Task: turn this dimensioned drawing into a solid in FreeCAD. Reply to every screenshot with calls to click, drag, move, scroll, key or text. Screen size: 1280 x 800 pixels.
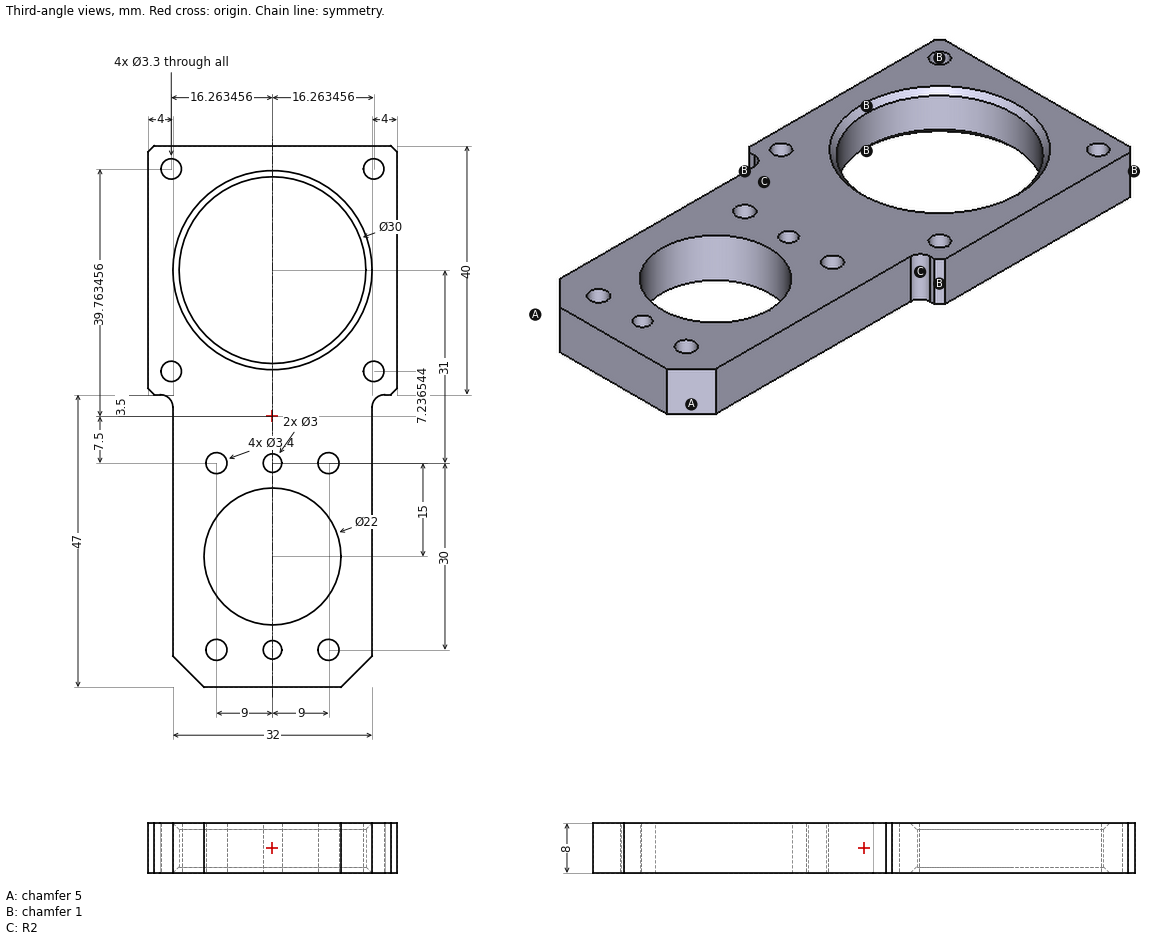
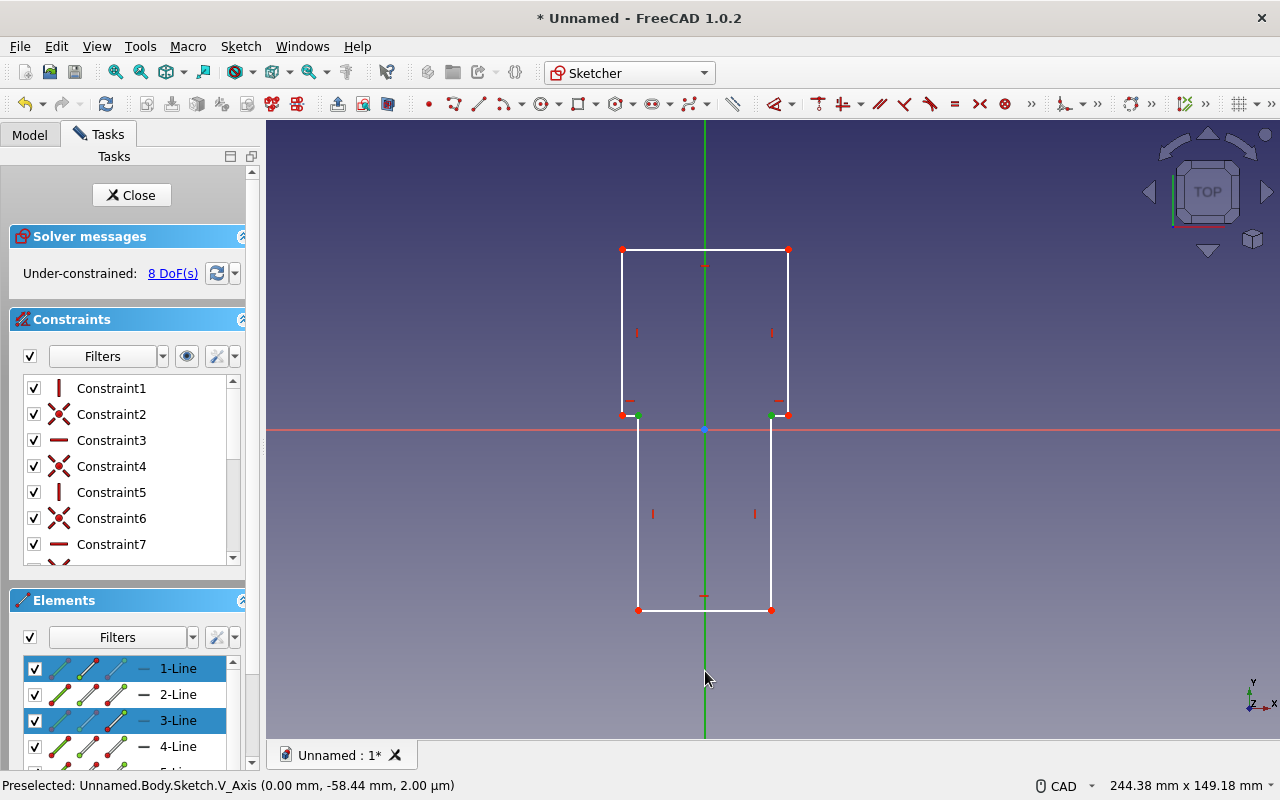
click(980, 104)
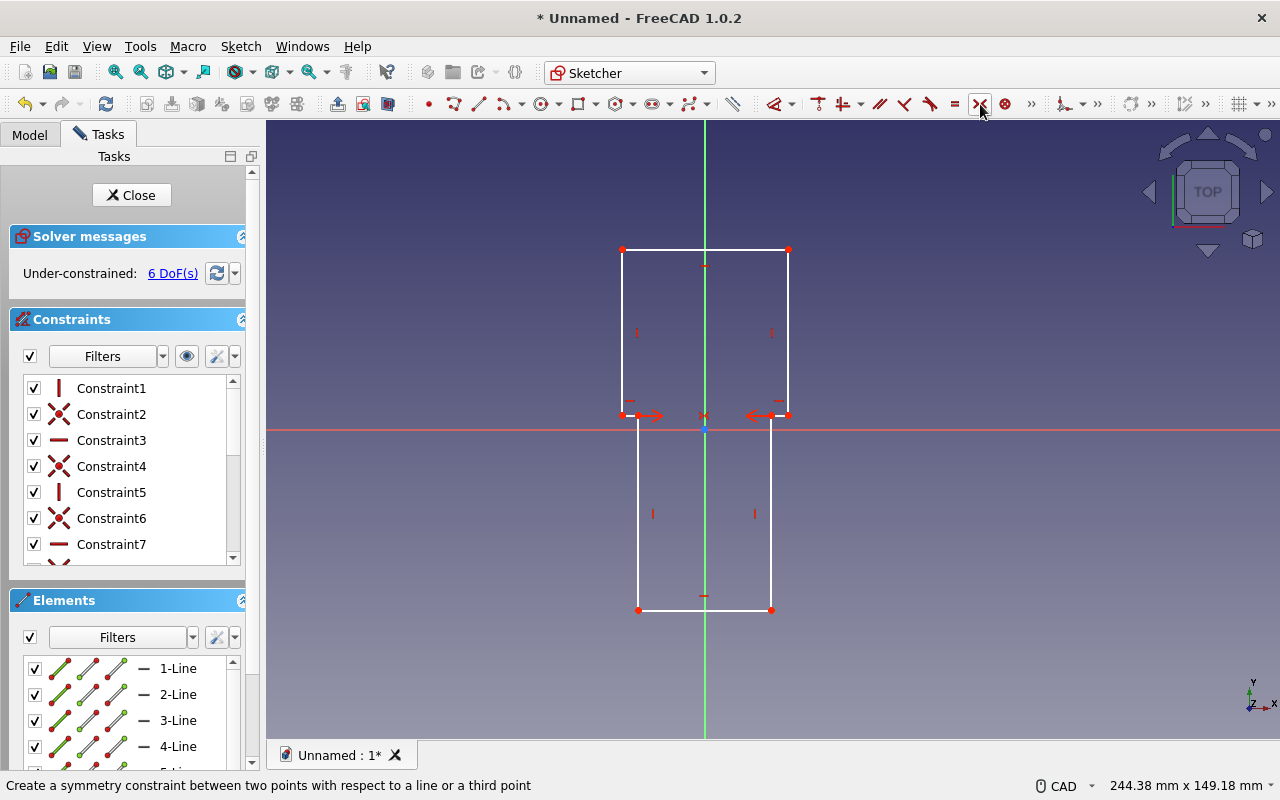
key(d)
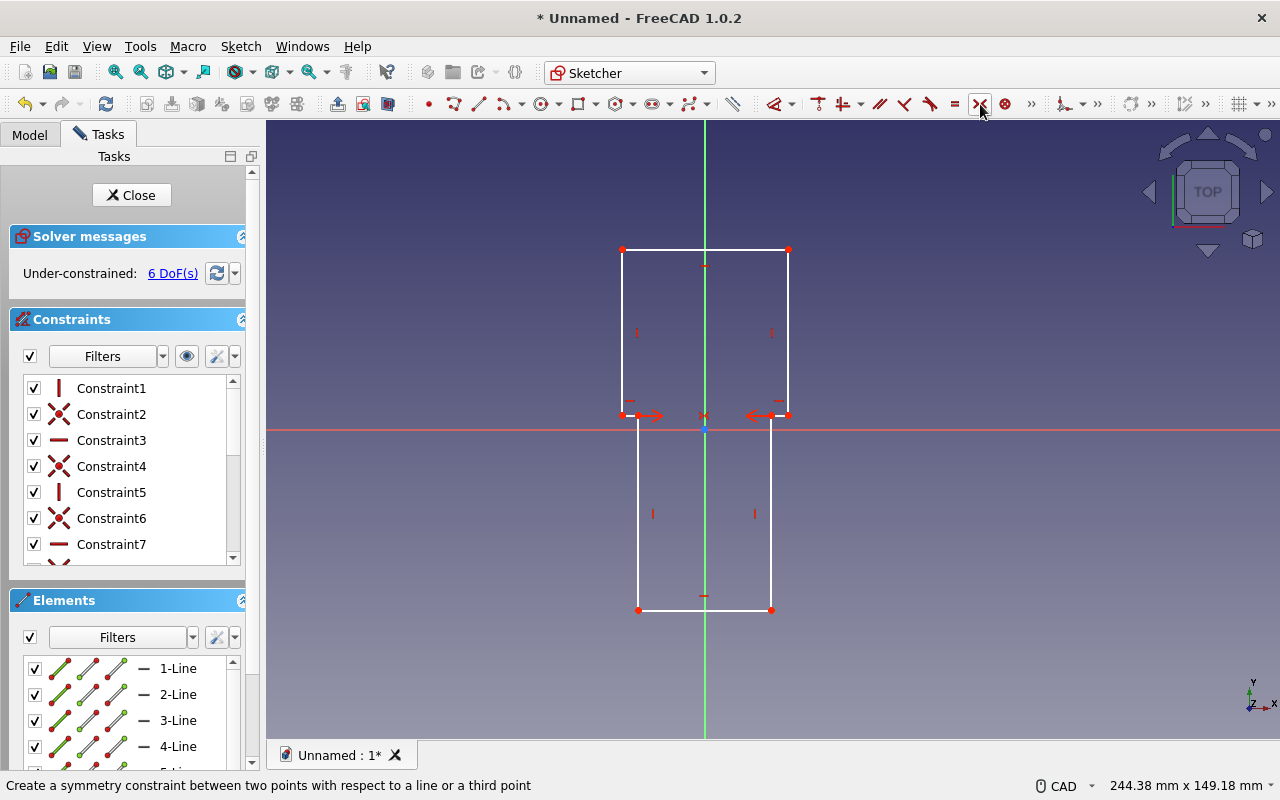
scroll(780, 416, up, 5)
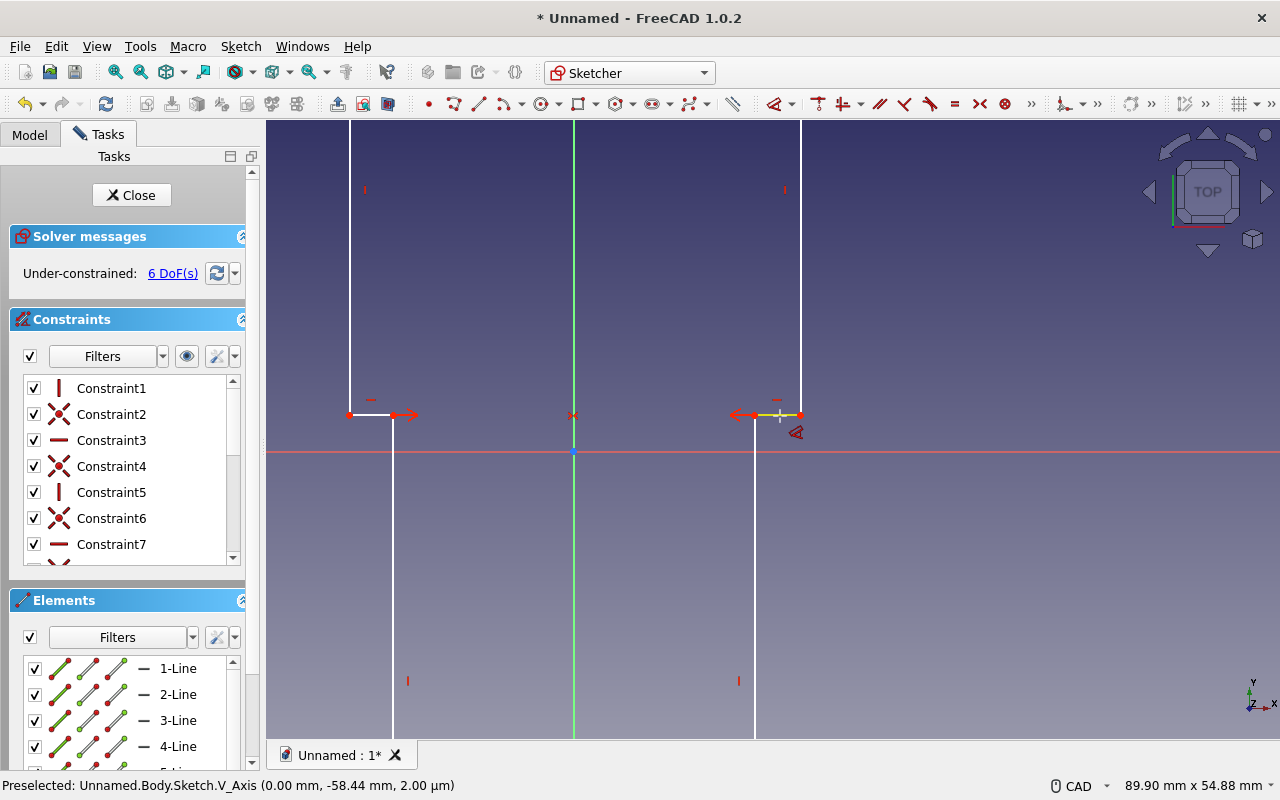
click(778, 415)
click(778, 381)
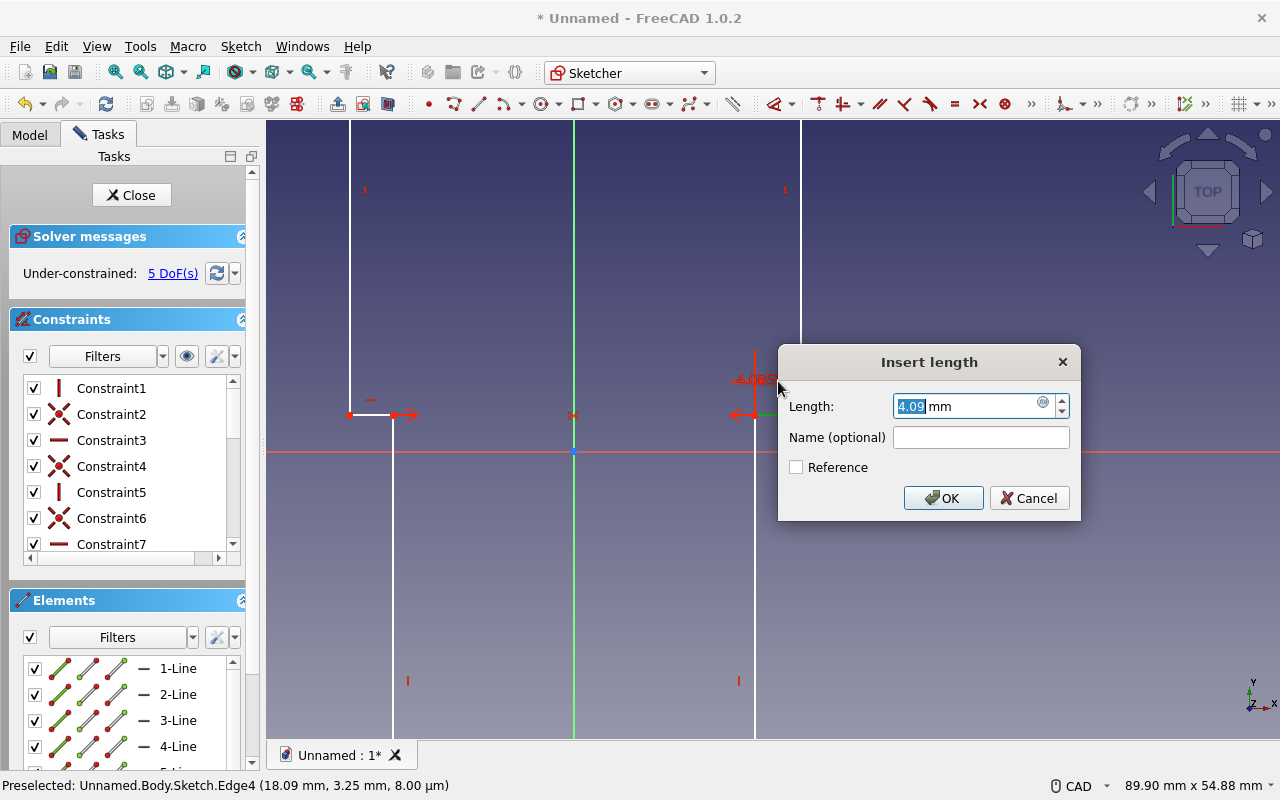
text(4)
key(Return)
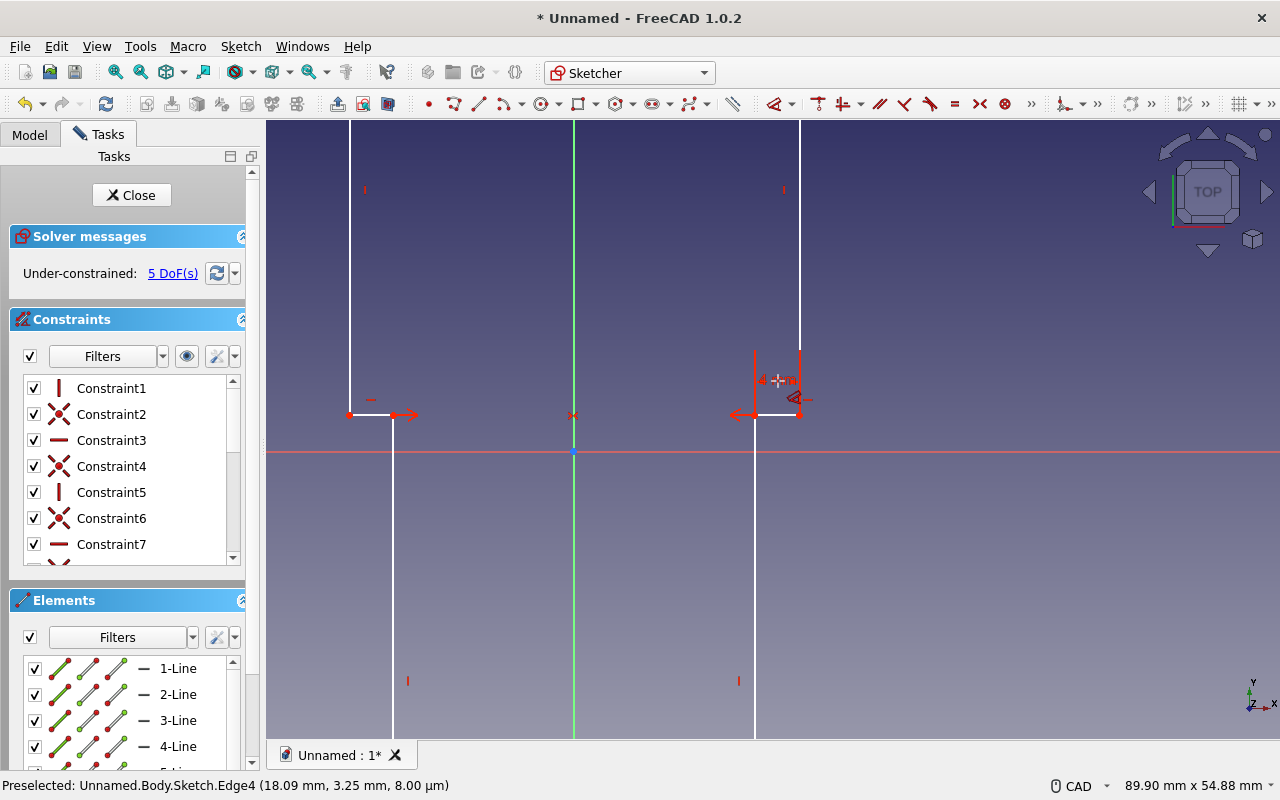
click(363, 415)
click(371, 381)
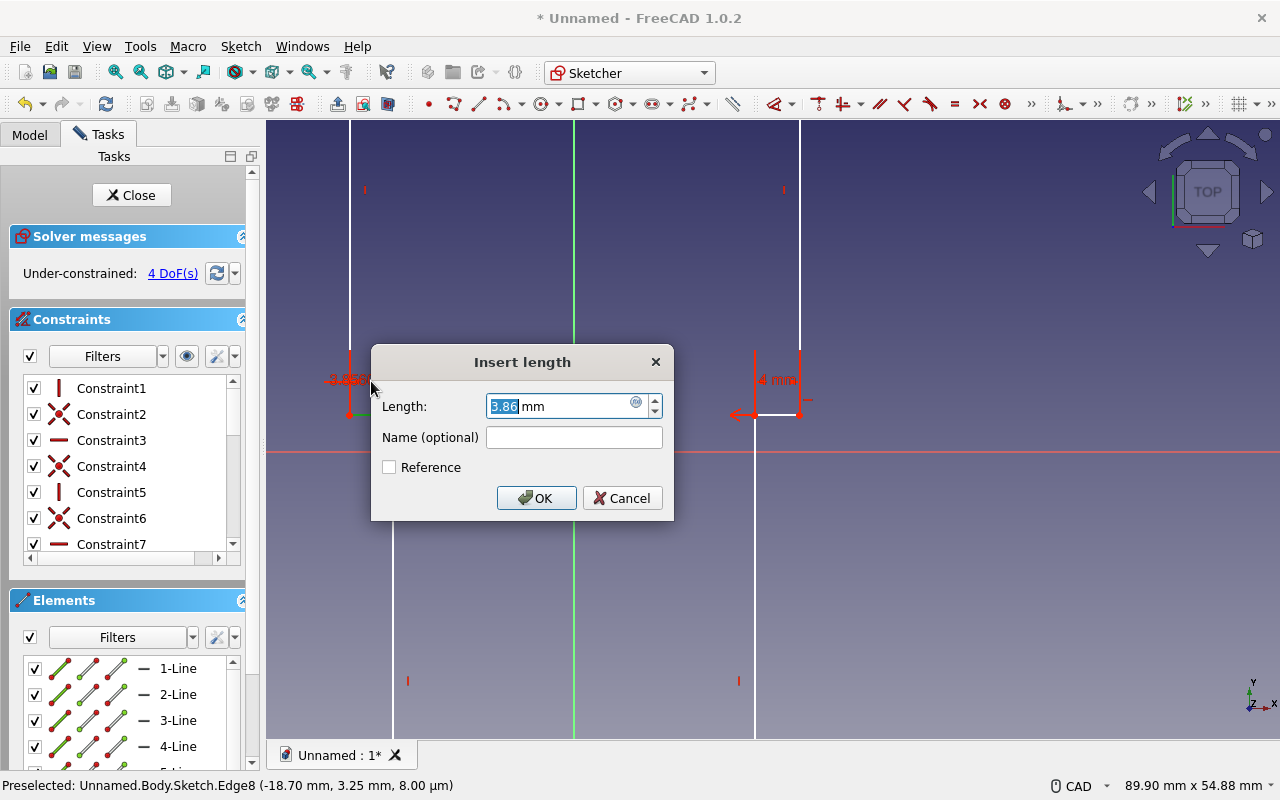
text(4)
key(Return)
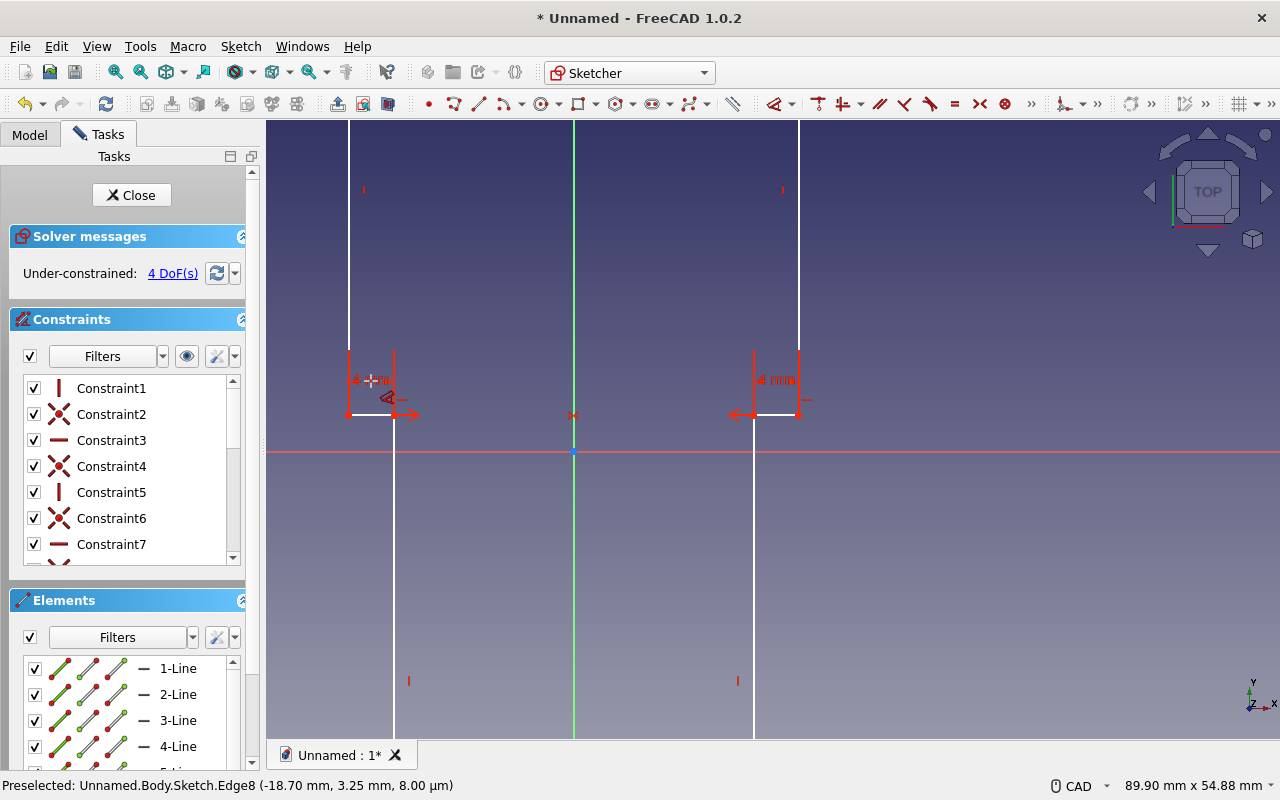
click(394, 574)
click(360, 563)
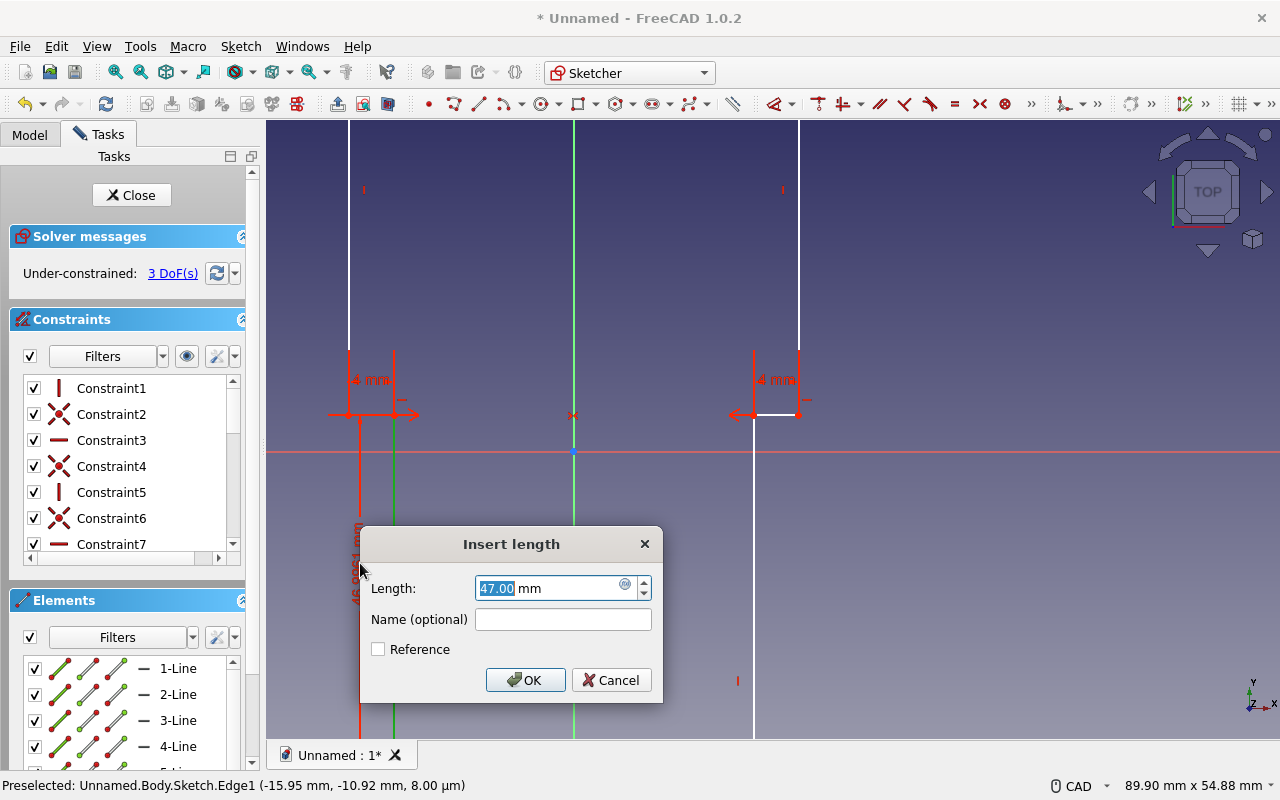
text(47)
key(Return)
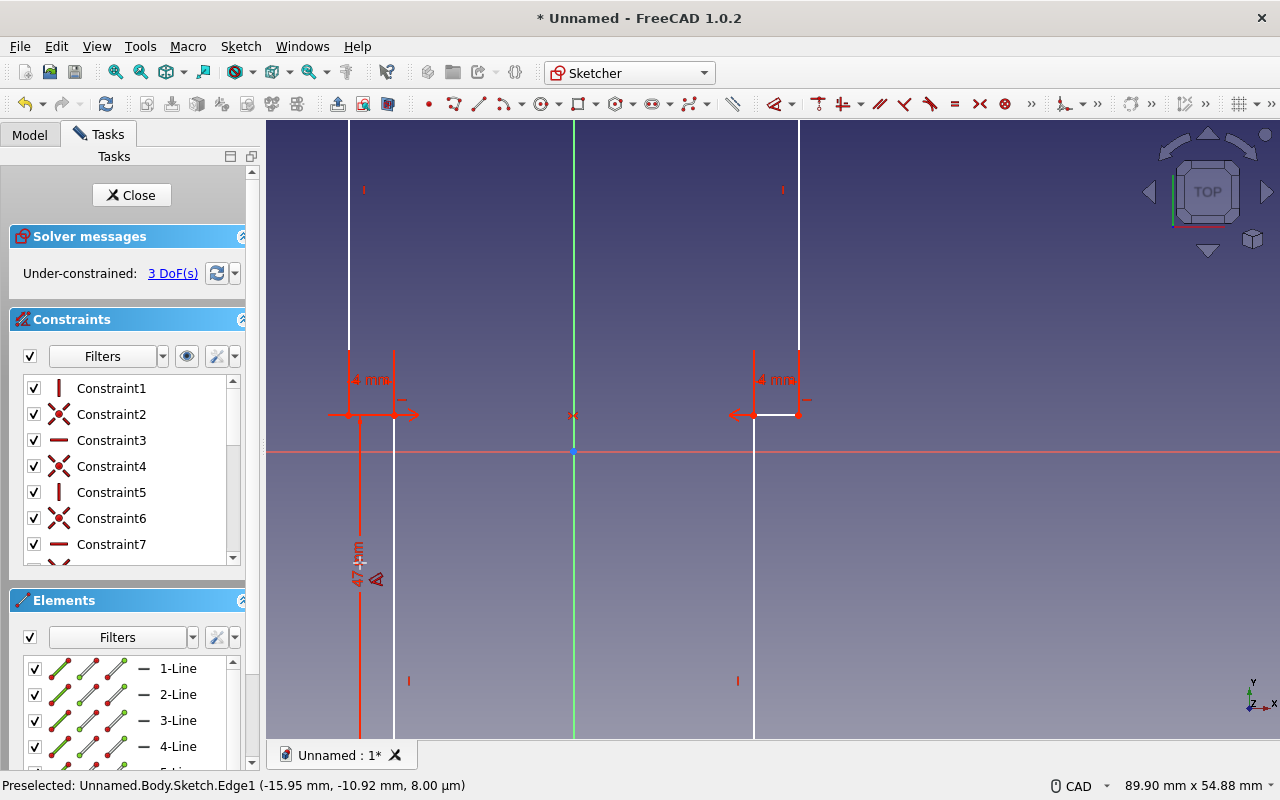
scroll(780, 416, down, 5)